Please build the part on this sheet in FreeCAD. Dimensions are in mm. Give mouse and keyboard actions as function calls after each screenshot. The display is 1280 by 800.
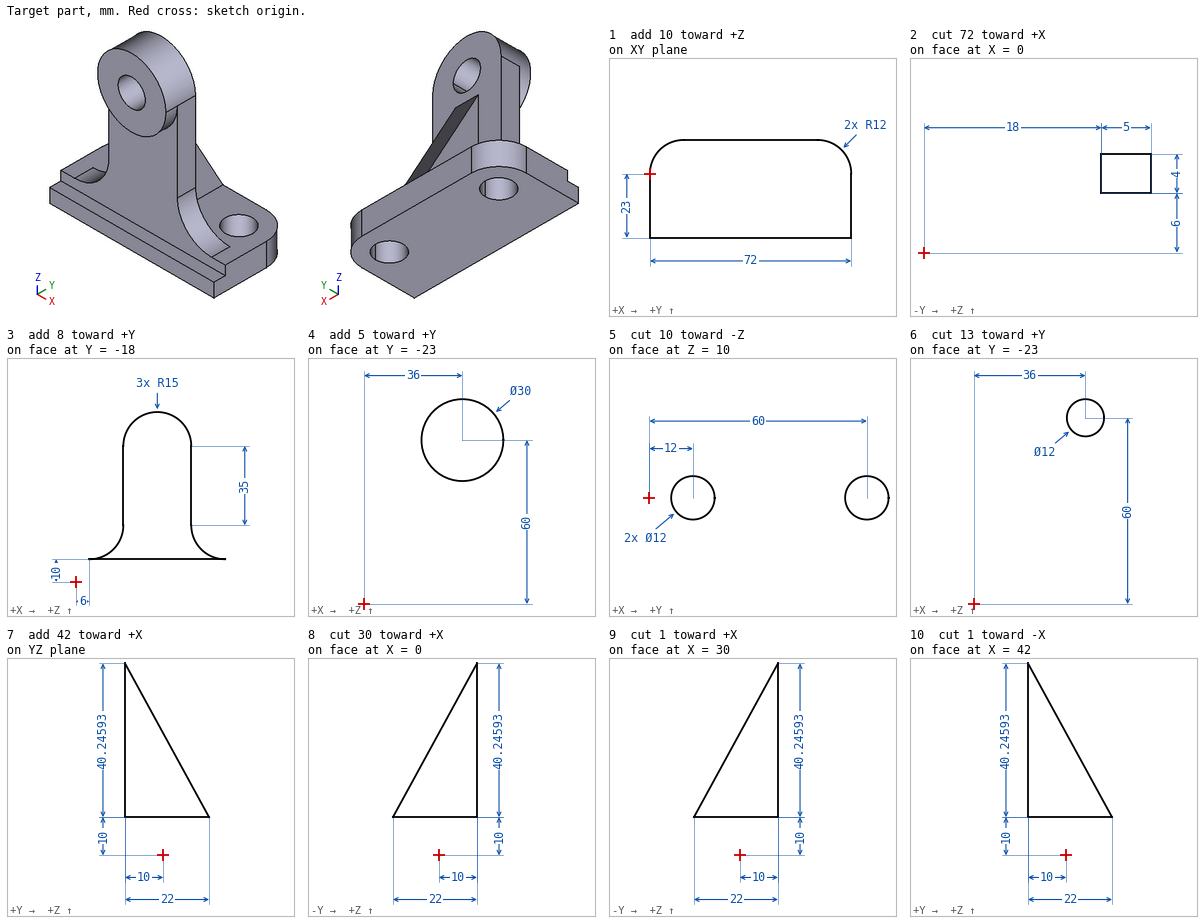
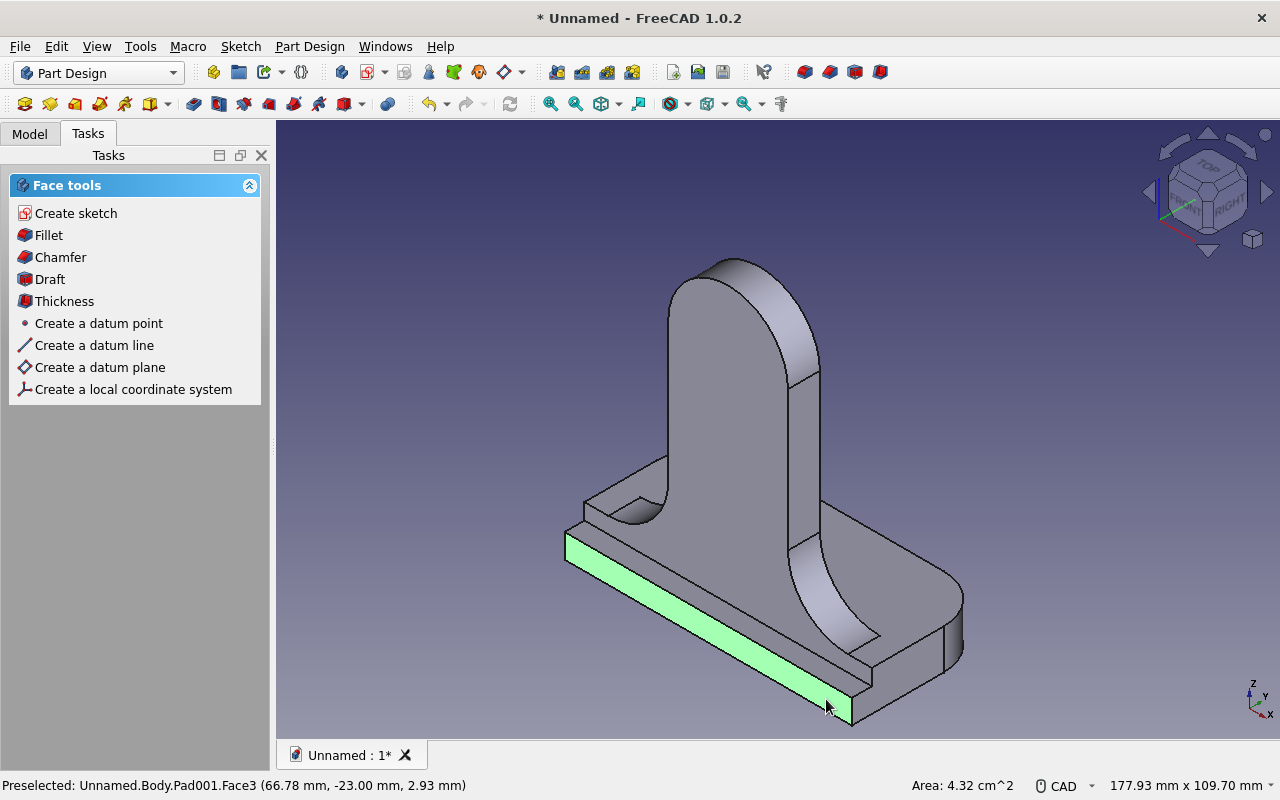
click(366, 72)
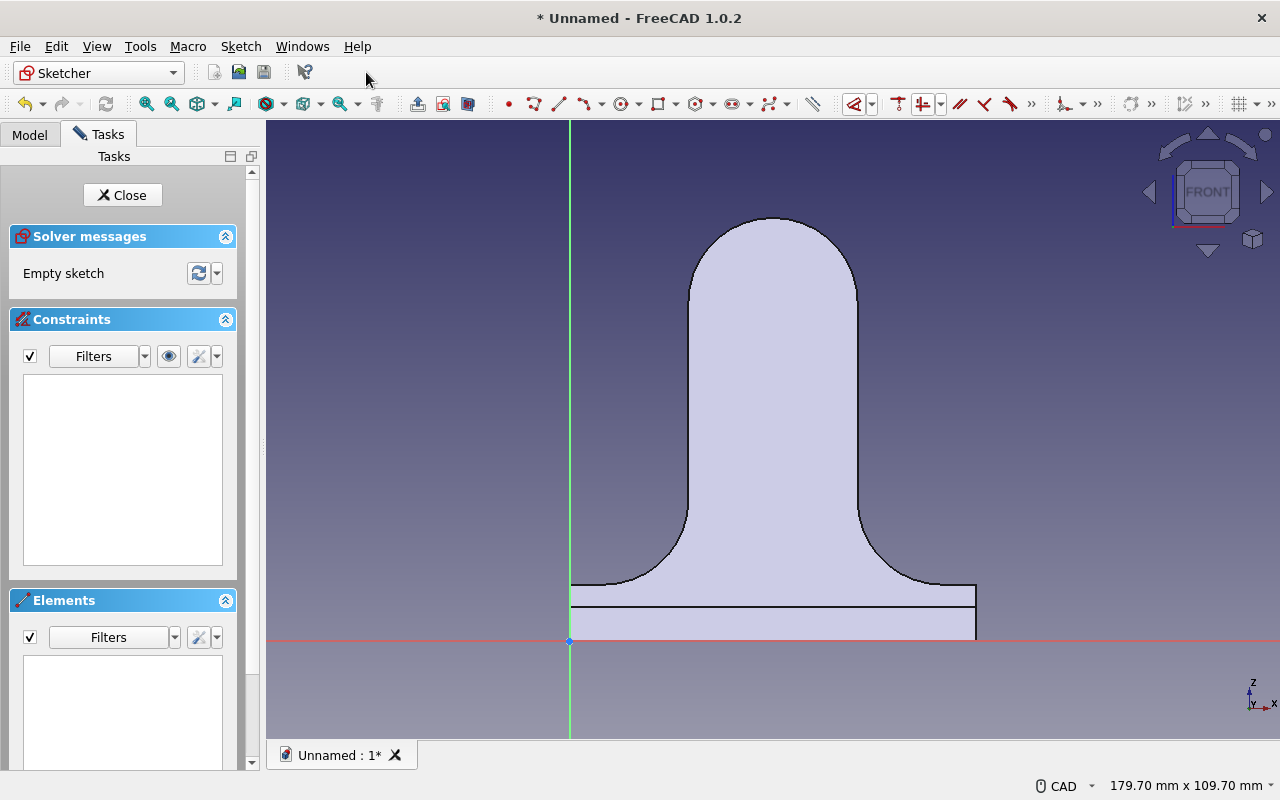
scroll(829, 199, up, 4)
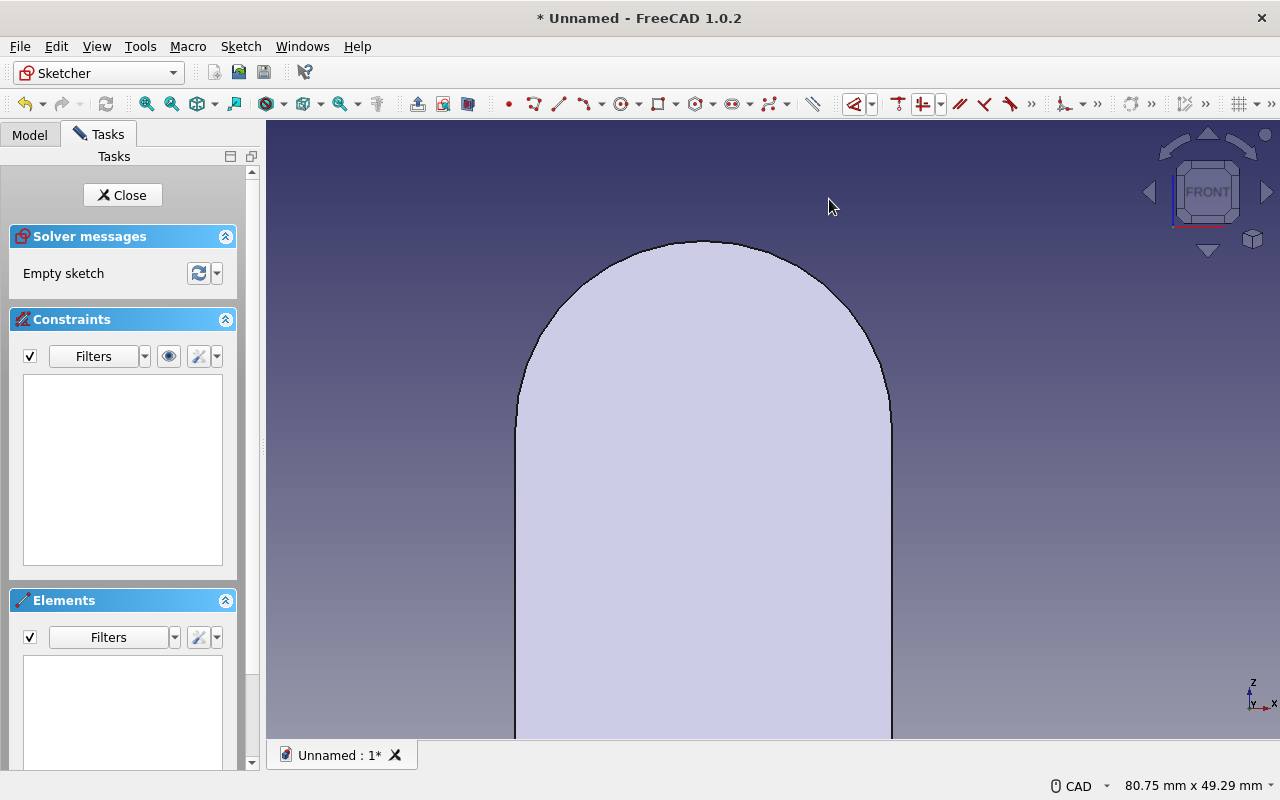
click(620, 104)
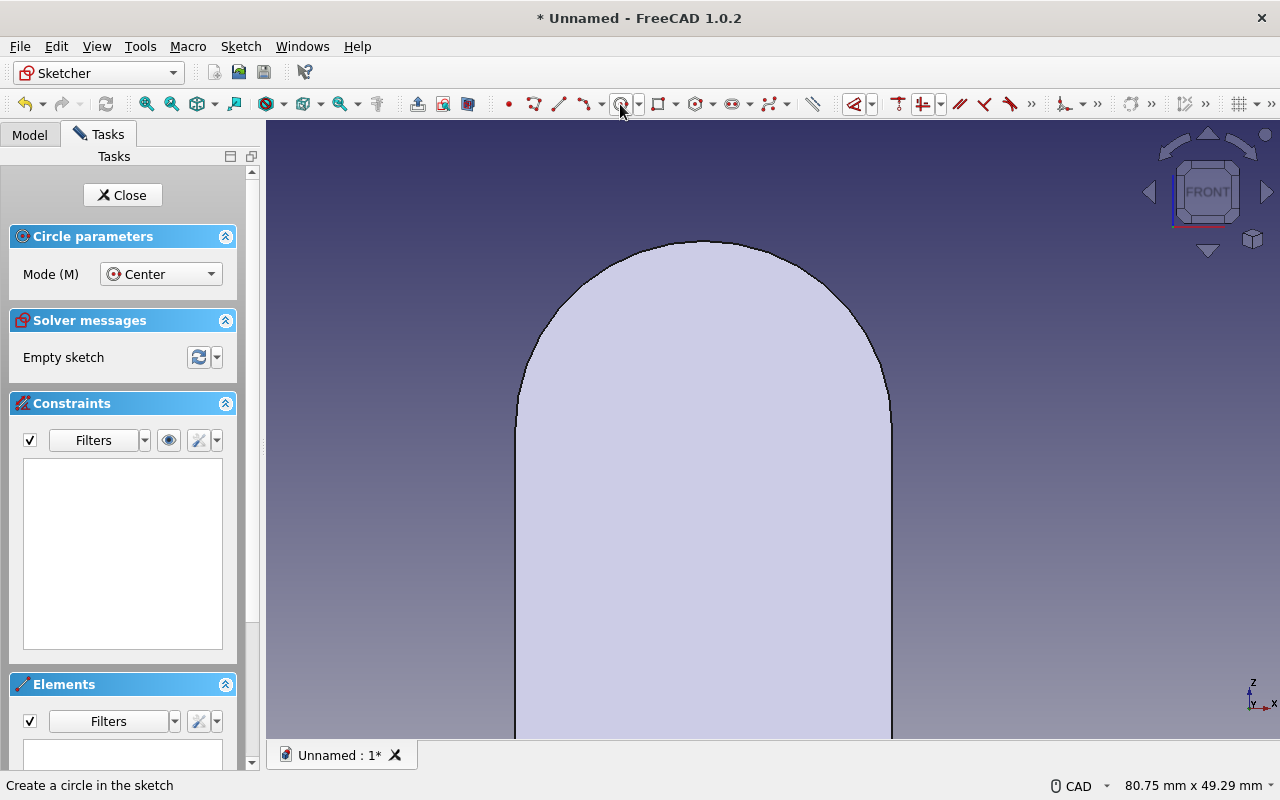
click(704, 429)
move(837, 296)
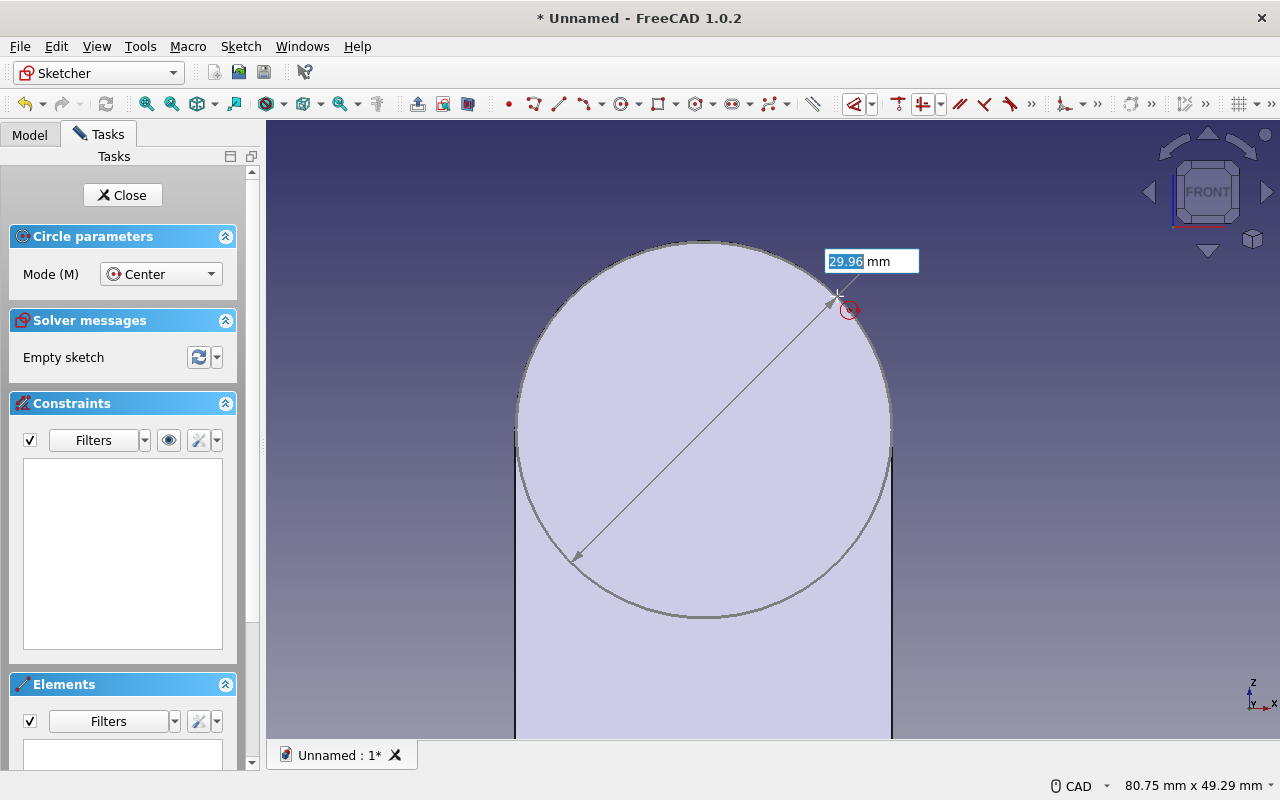
text(30)
key(Return)
key(Escape)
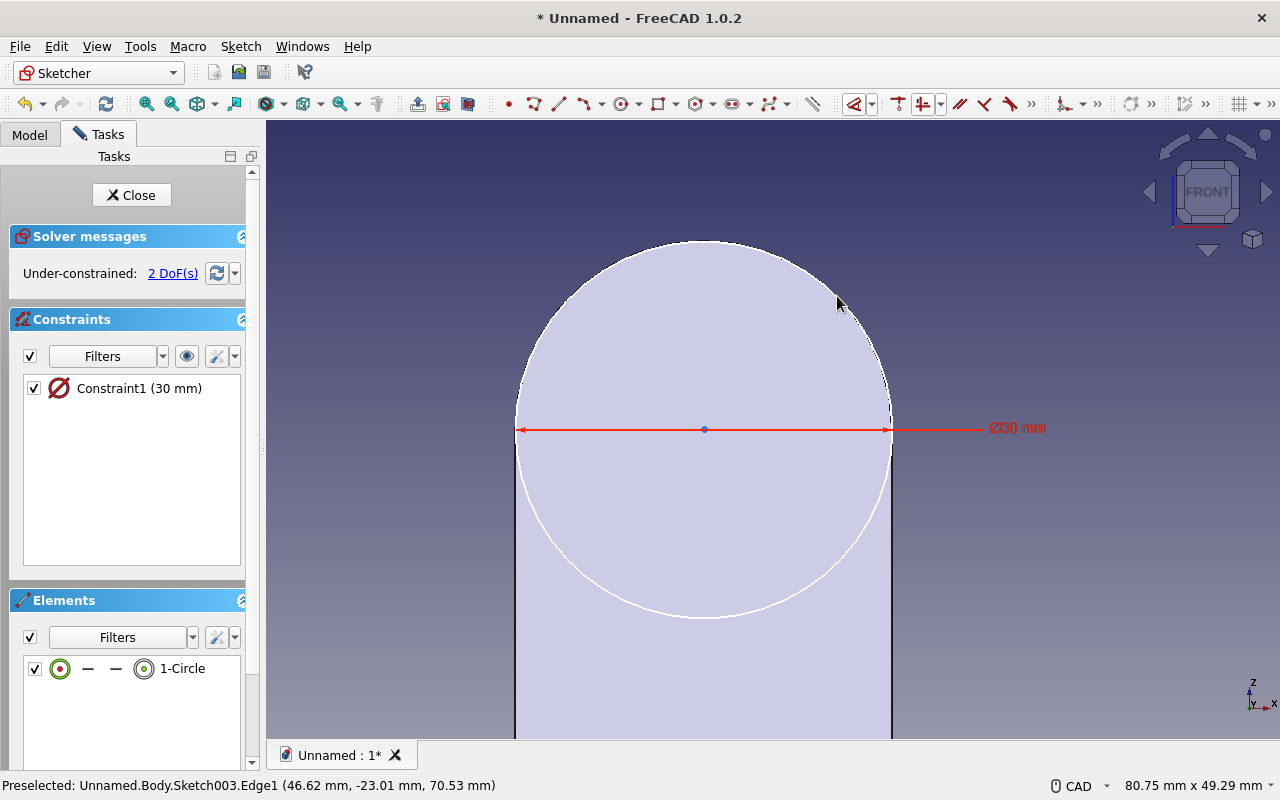
click(704, 430)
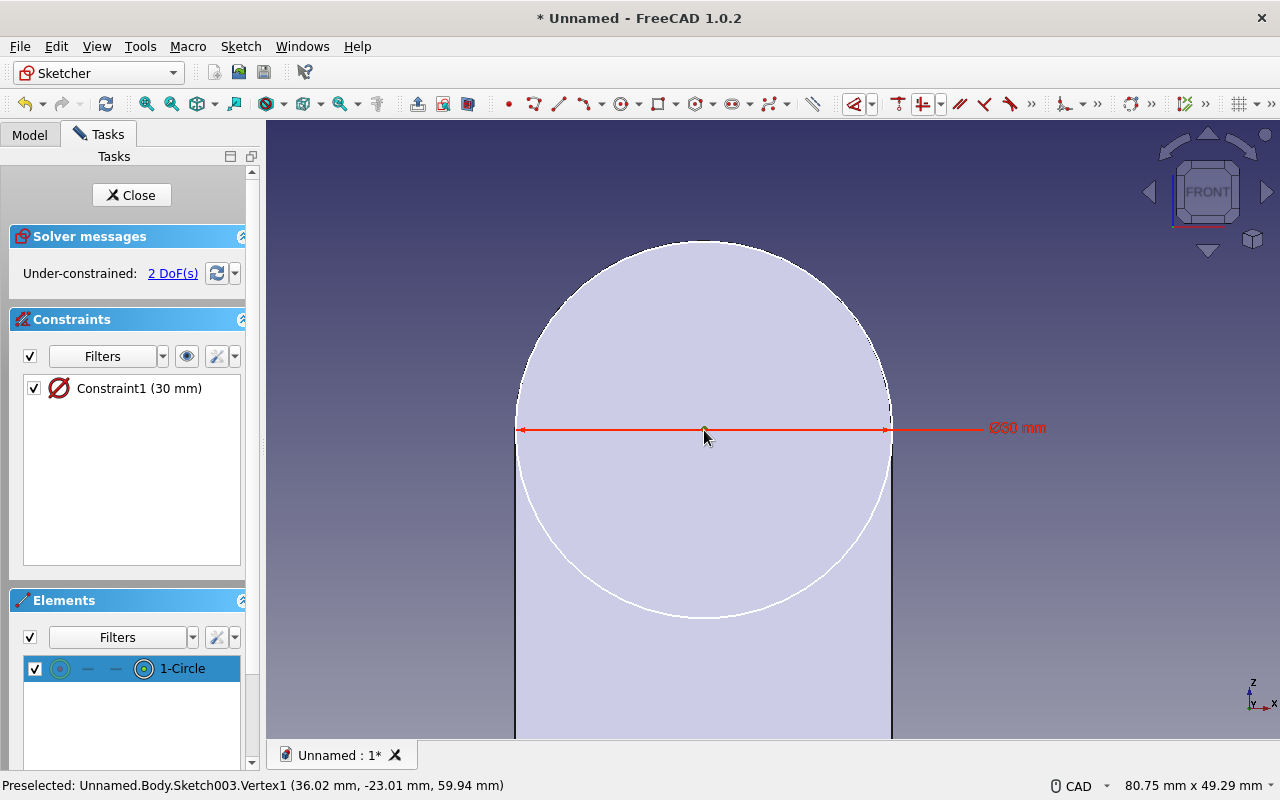
key(l)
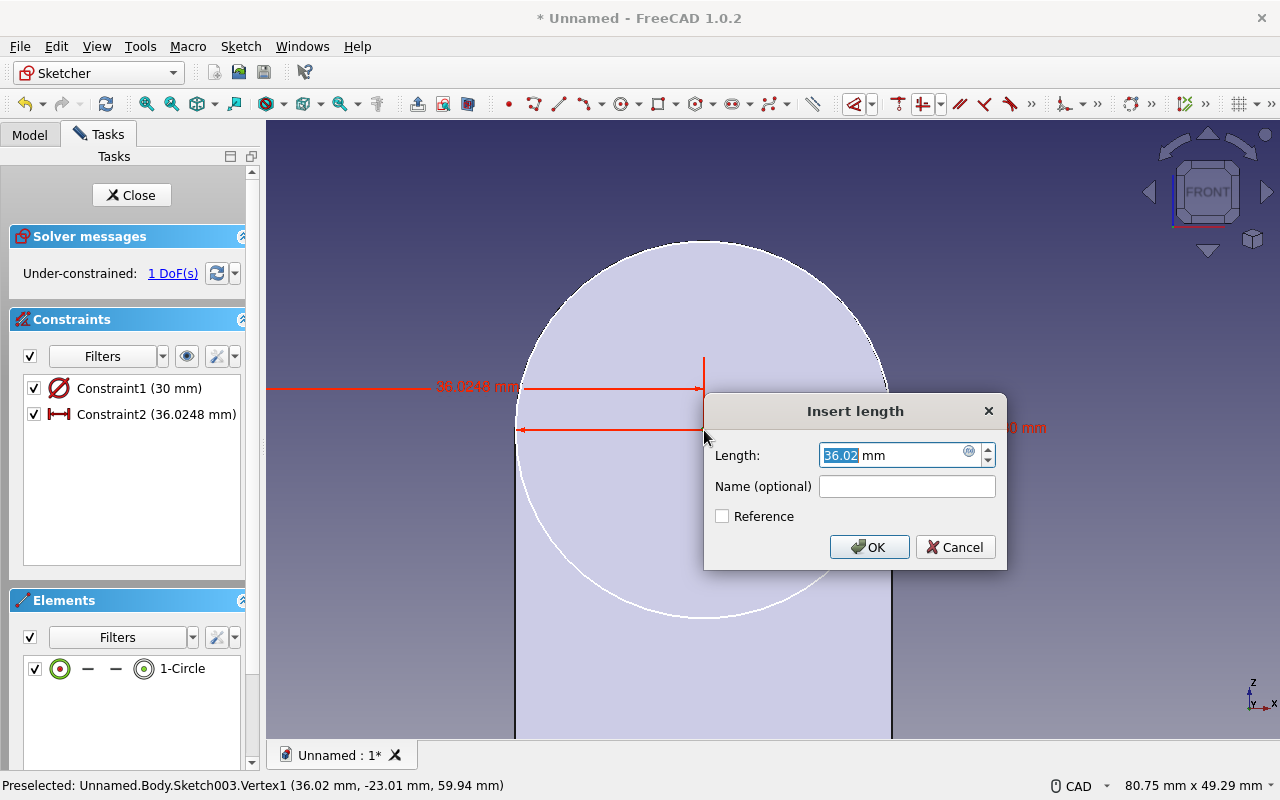
text(36)
key(Return)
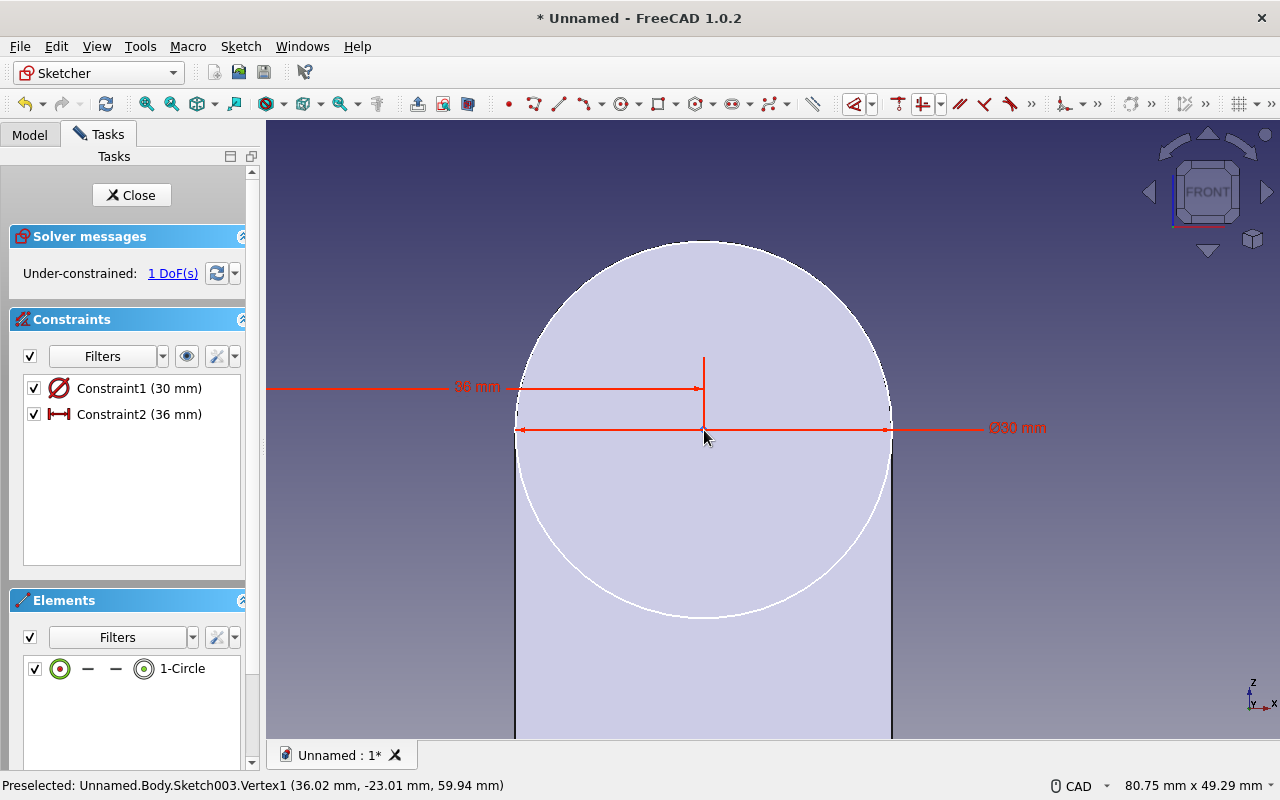
click(704, 430)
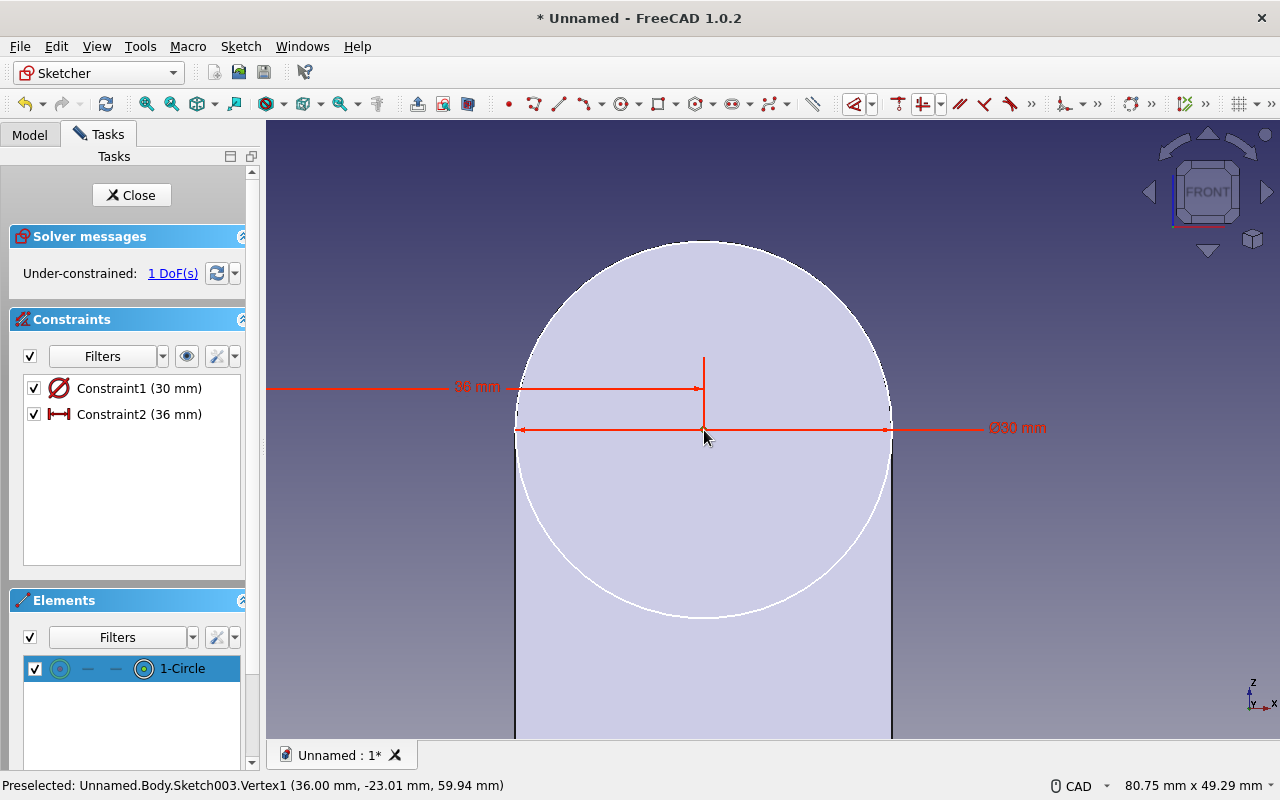
key(i)